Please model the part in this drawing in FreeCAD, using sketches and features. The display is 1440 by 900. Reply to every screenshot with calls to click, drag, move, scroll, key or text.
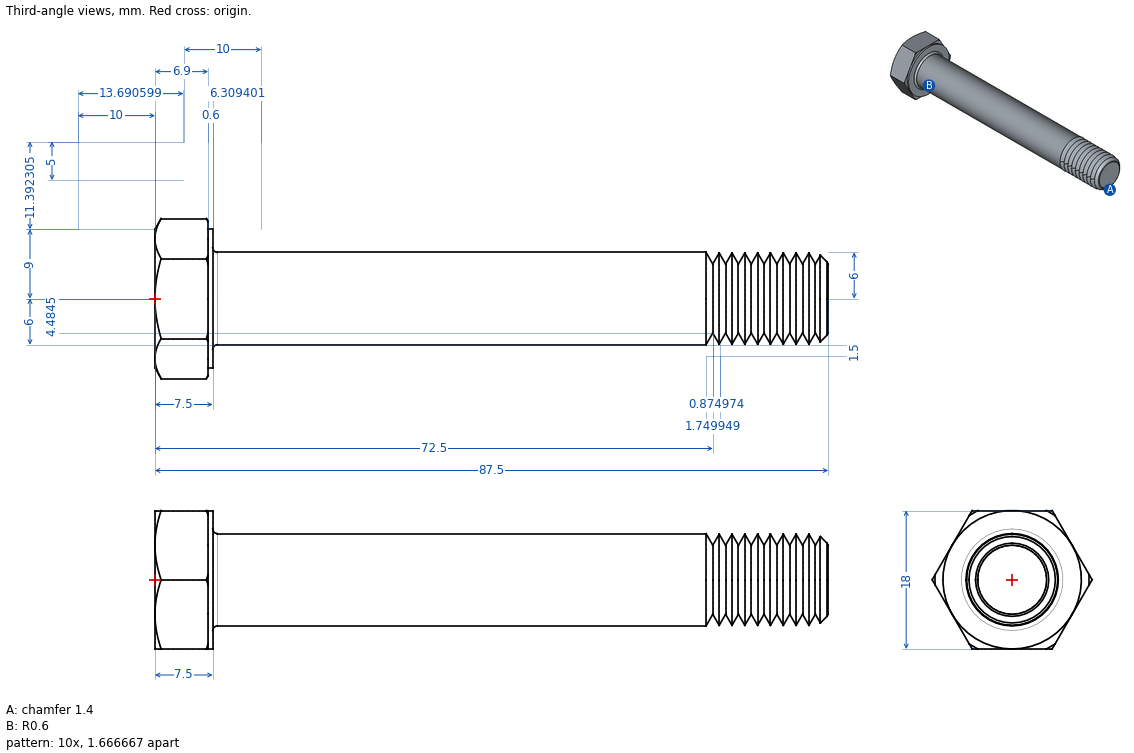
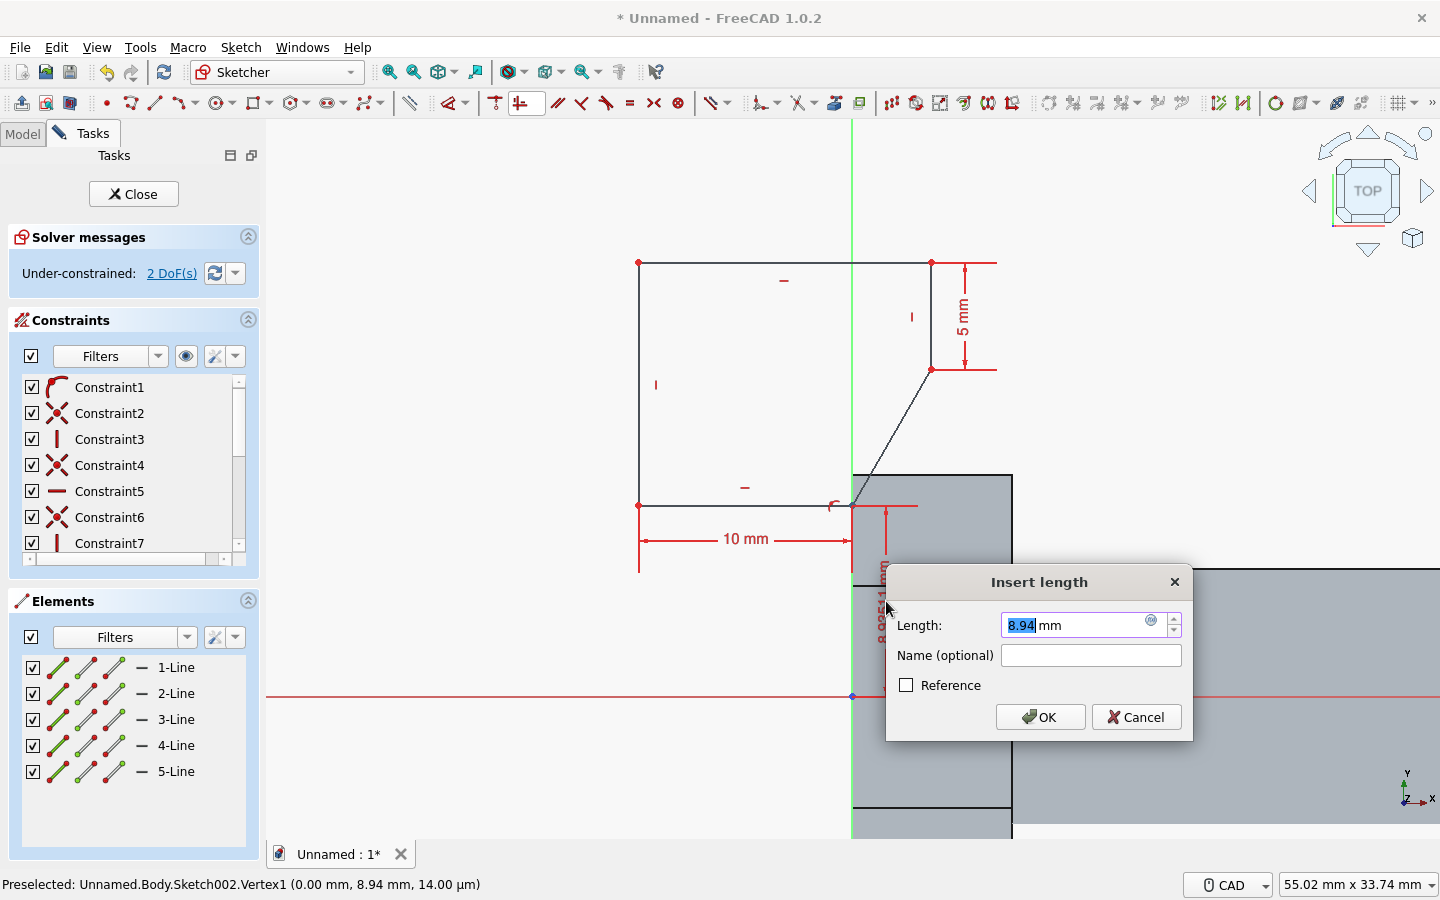
text(9)
key(Return)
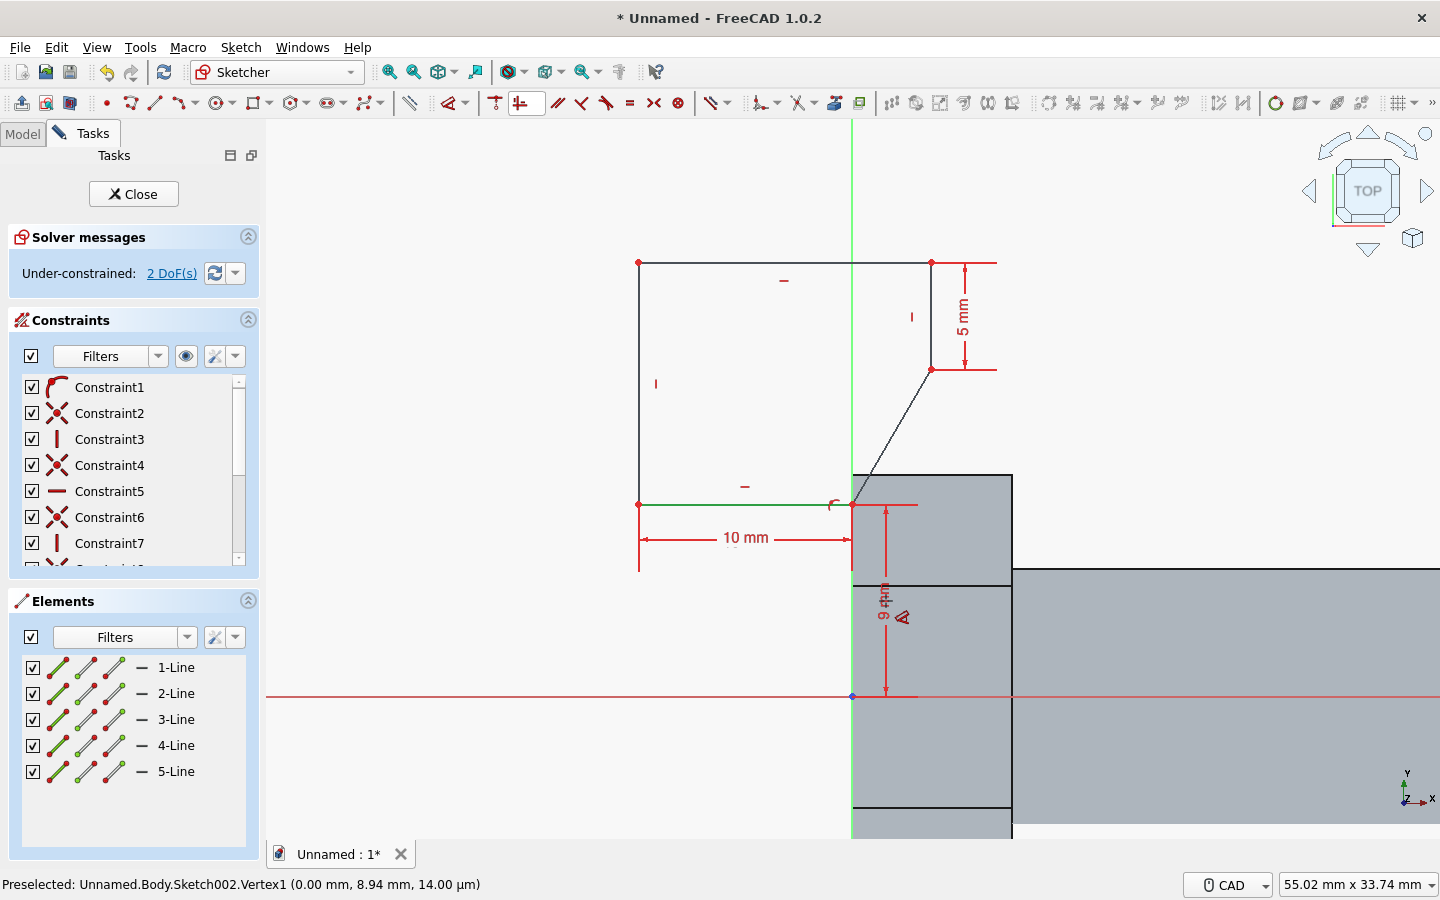
click(727, 263)
click(785, 229)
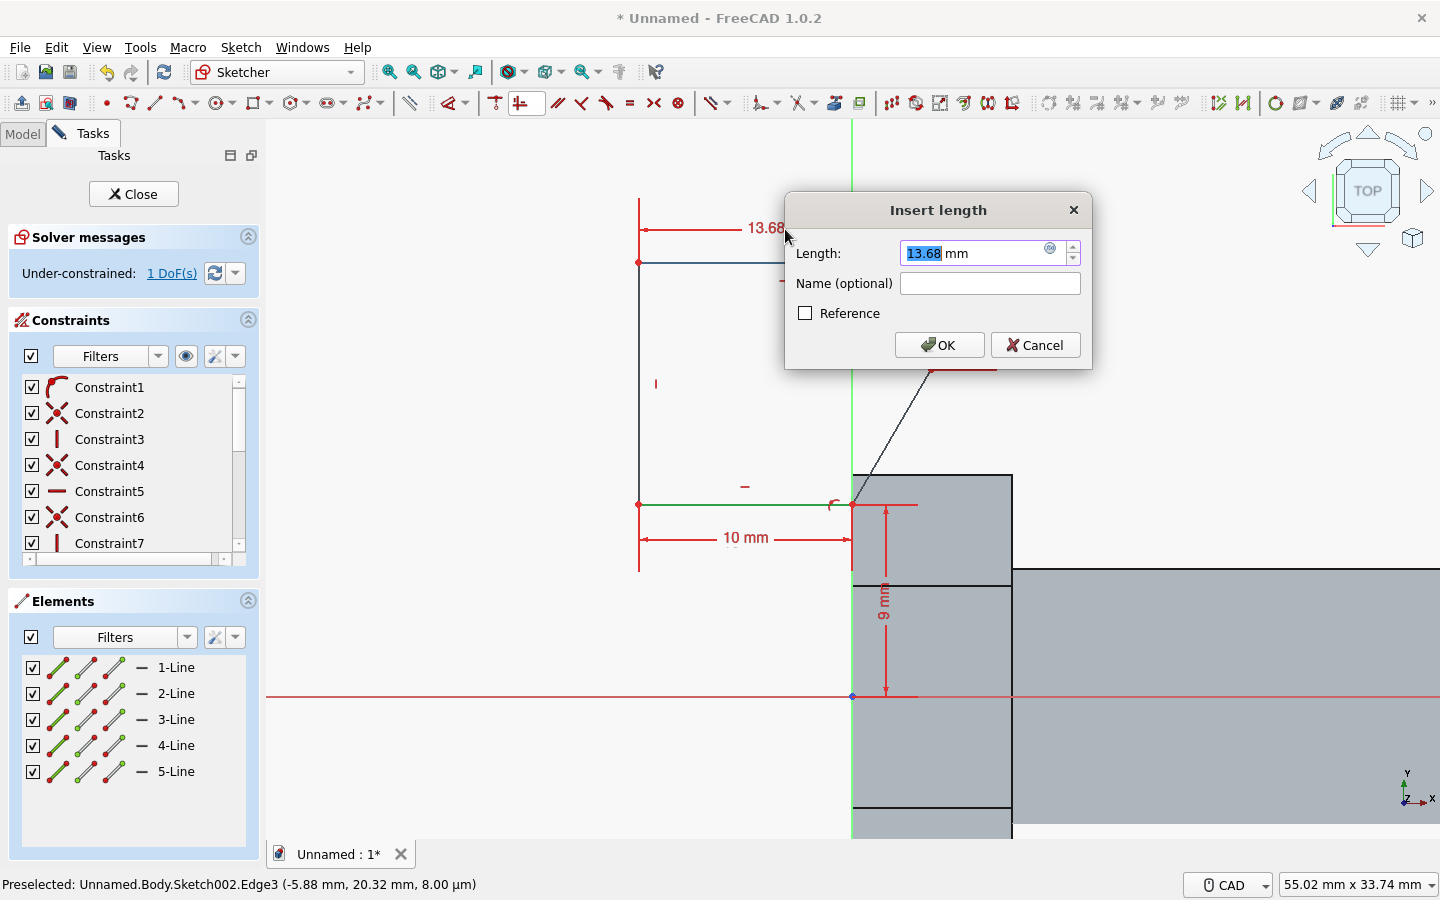
text(13.690599)
key(Return)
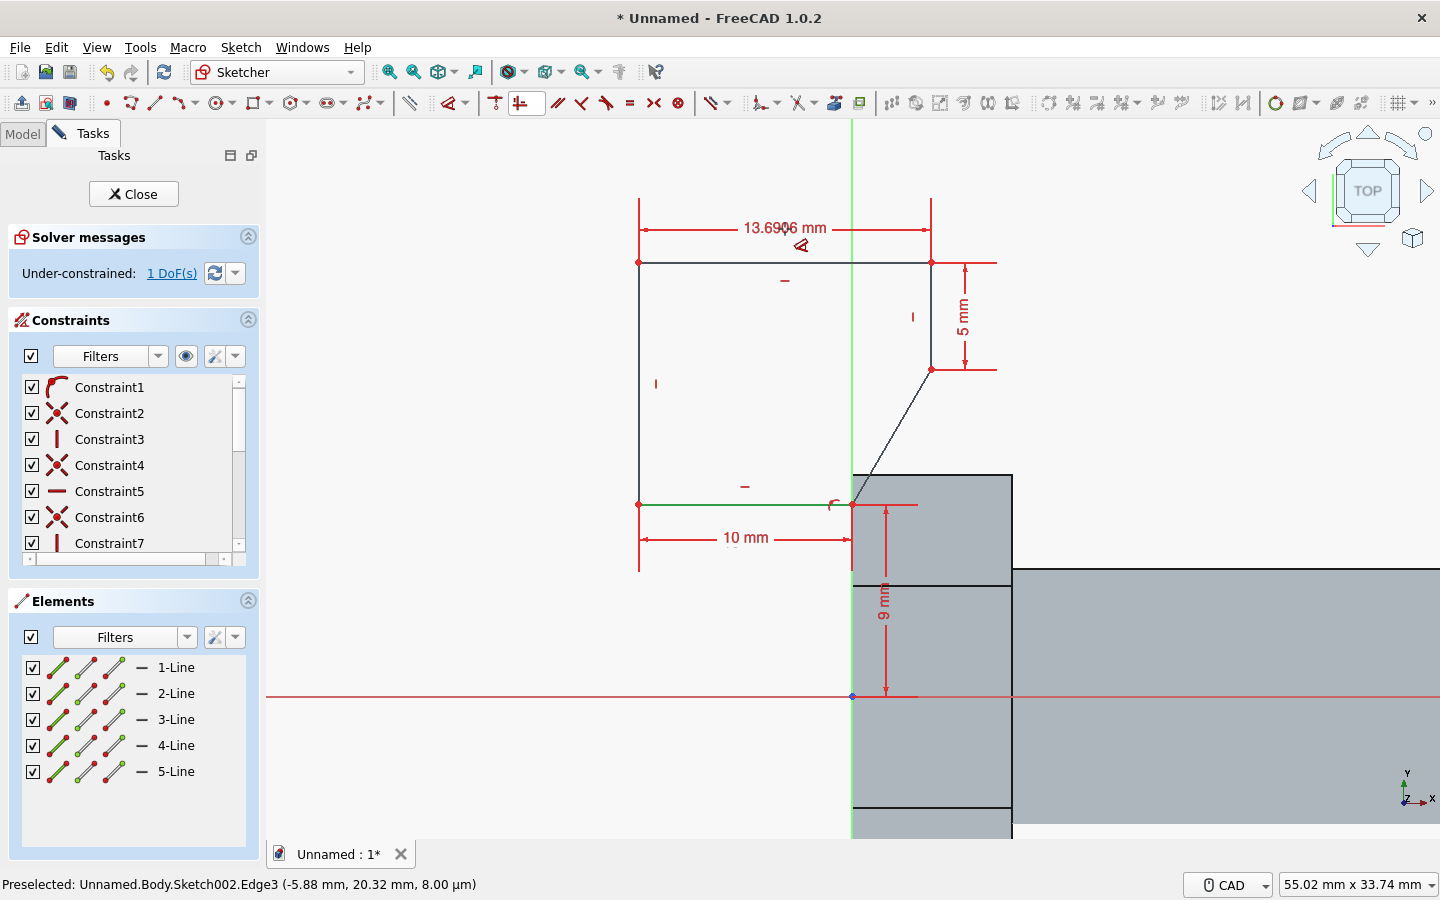
click(639, 335)
click(605, 384)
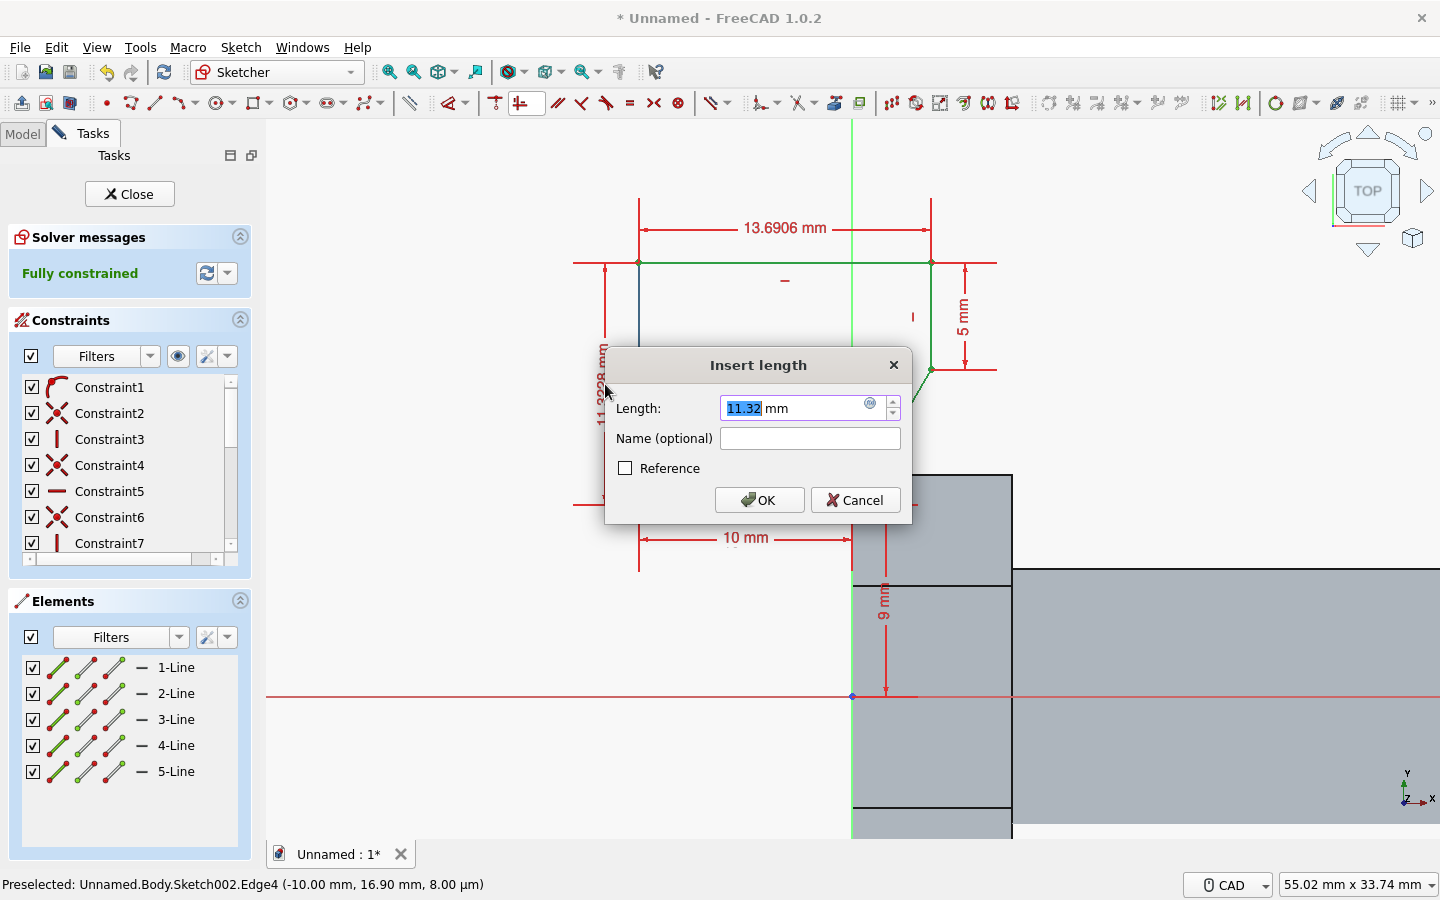
text(11.392305)
key(Return)
key(Escape)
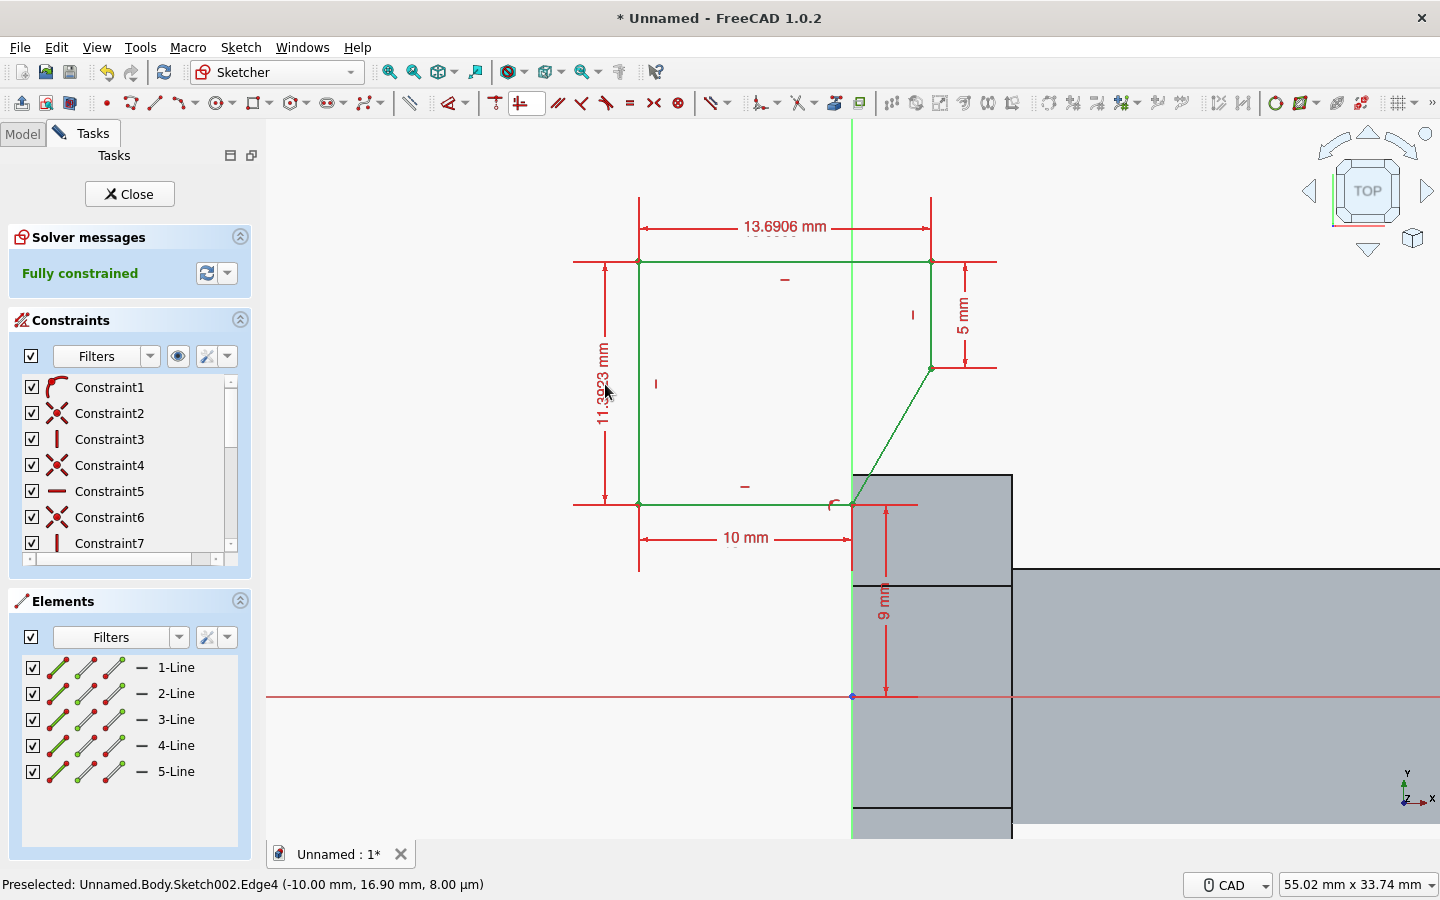
click(130, 194)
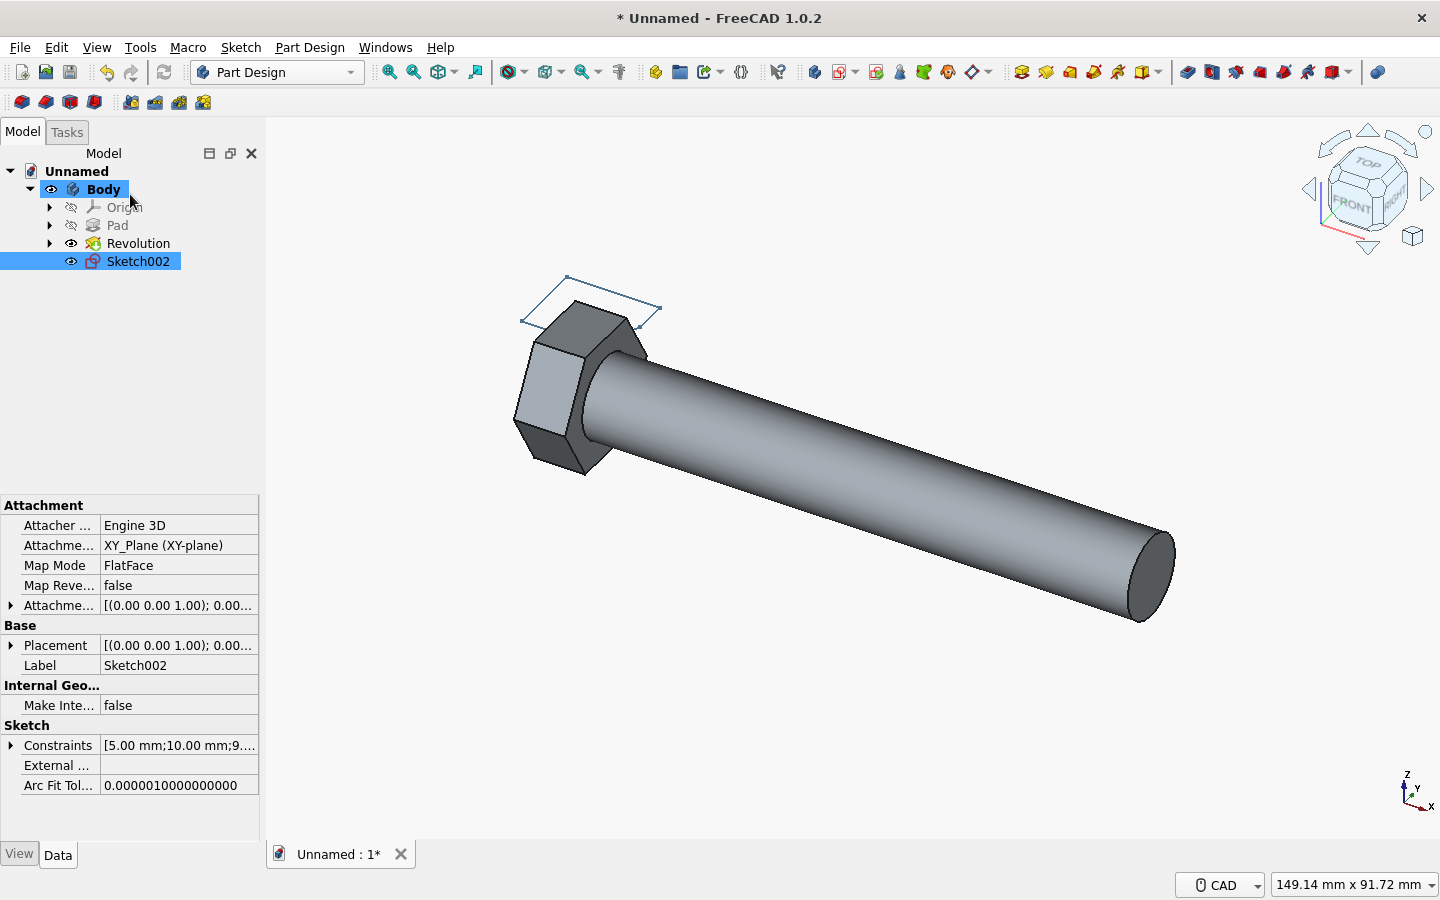
click(1236, 72)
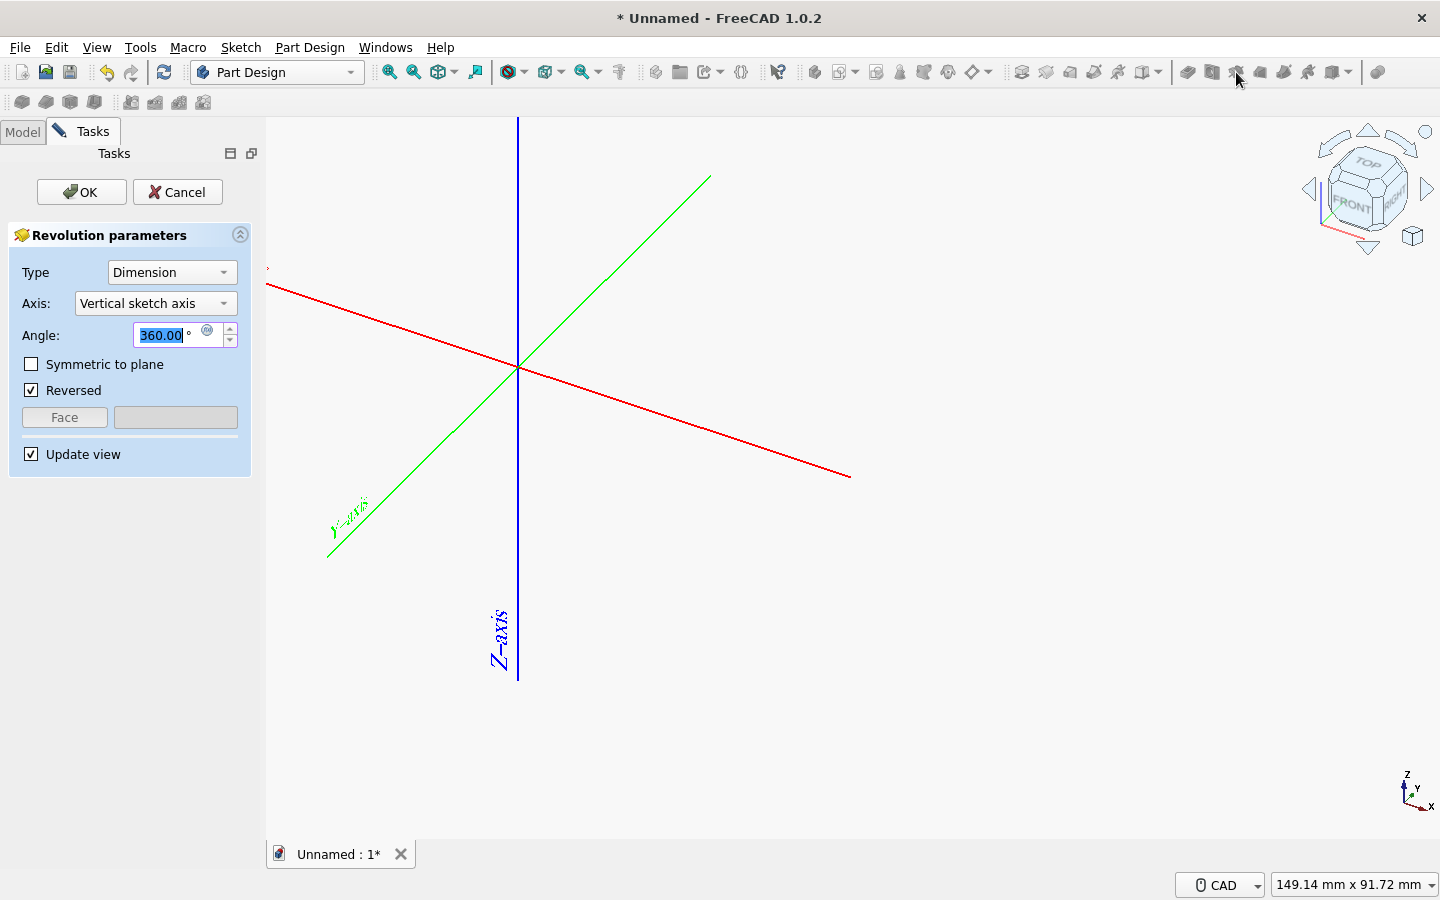
click(156, 304)